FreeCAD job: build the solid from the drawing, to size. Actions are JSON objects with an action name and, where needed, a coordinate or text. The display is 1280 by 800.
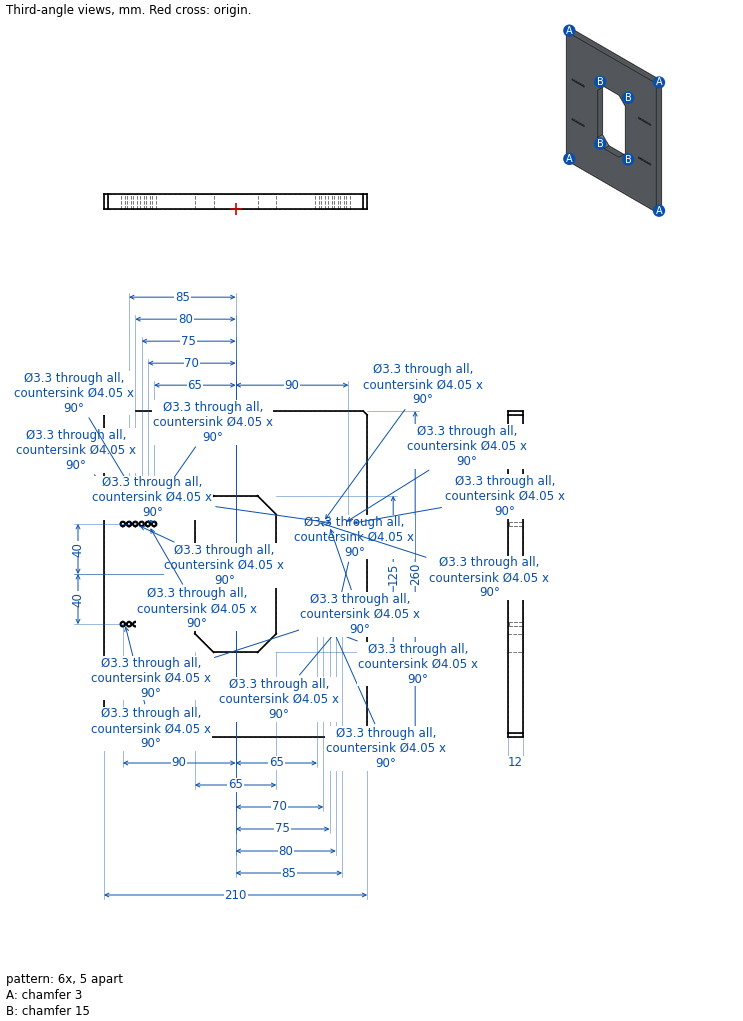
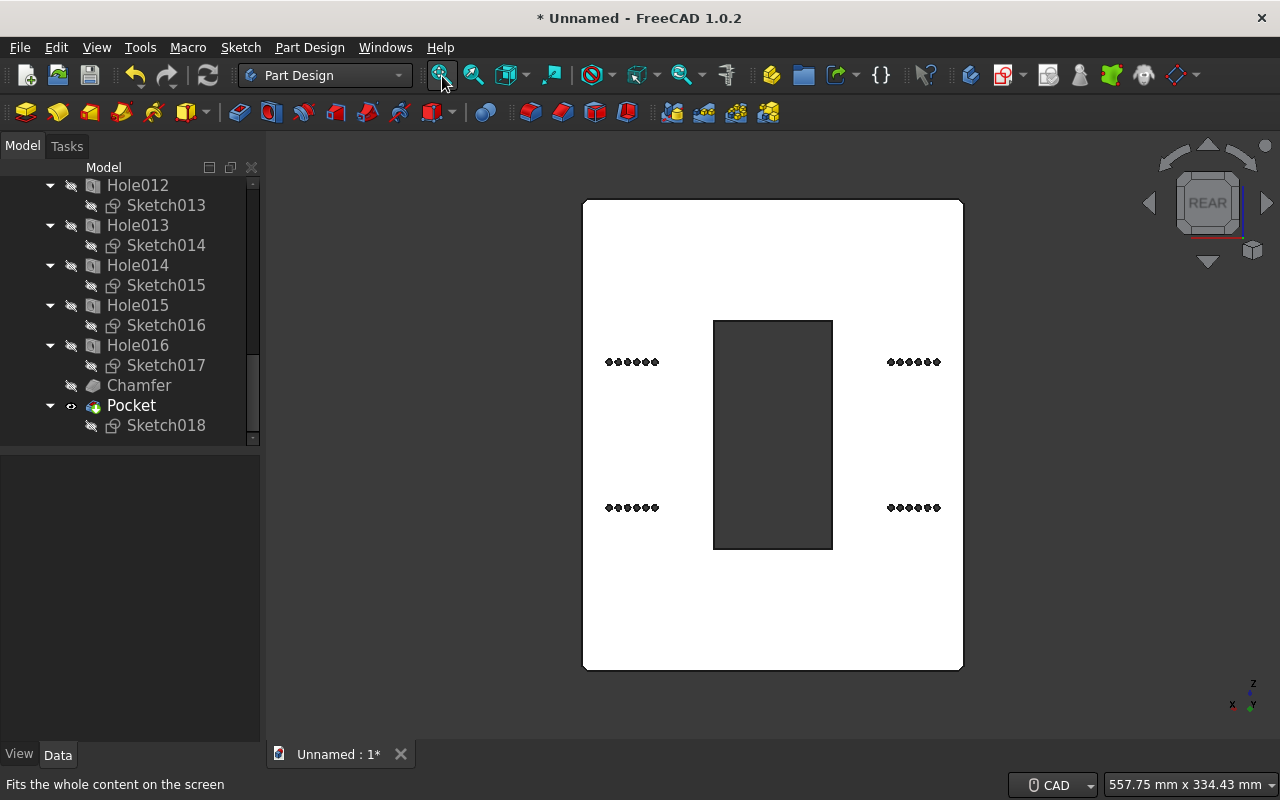
{"action": "scroll", "coordinate": [832, 548], "scroll_direction": "up", "scroll_amount": 4}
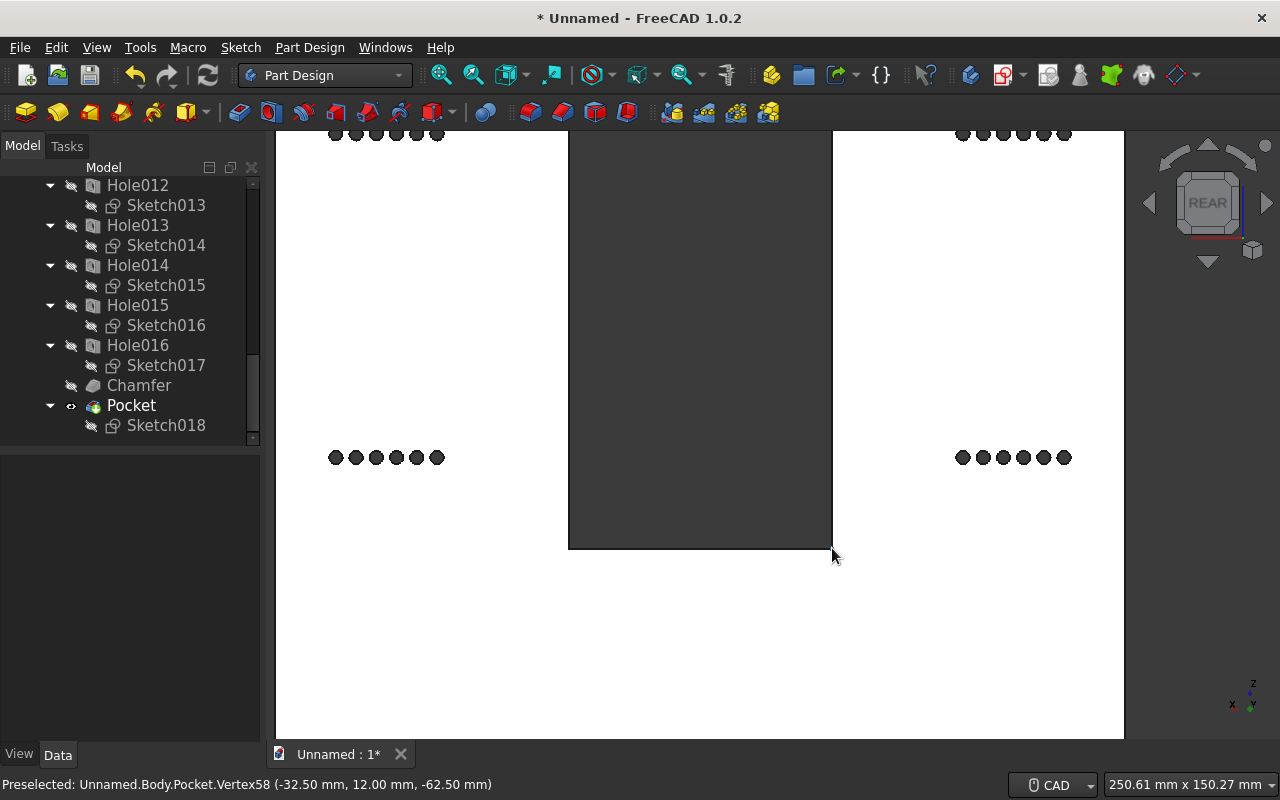
{"action": "left_click", "coordinate": [442, 76]}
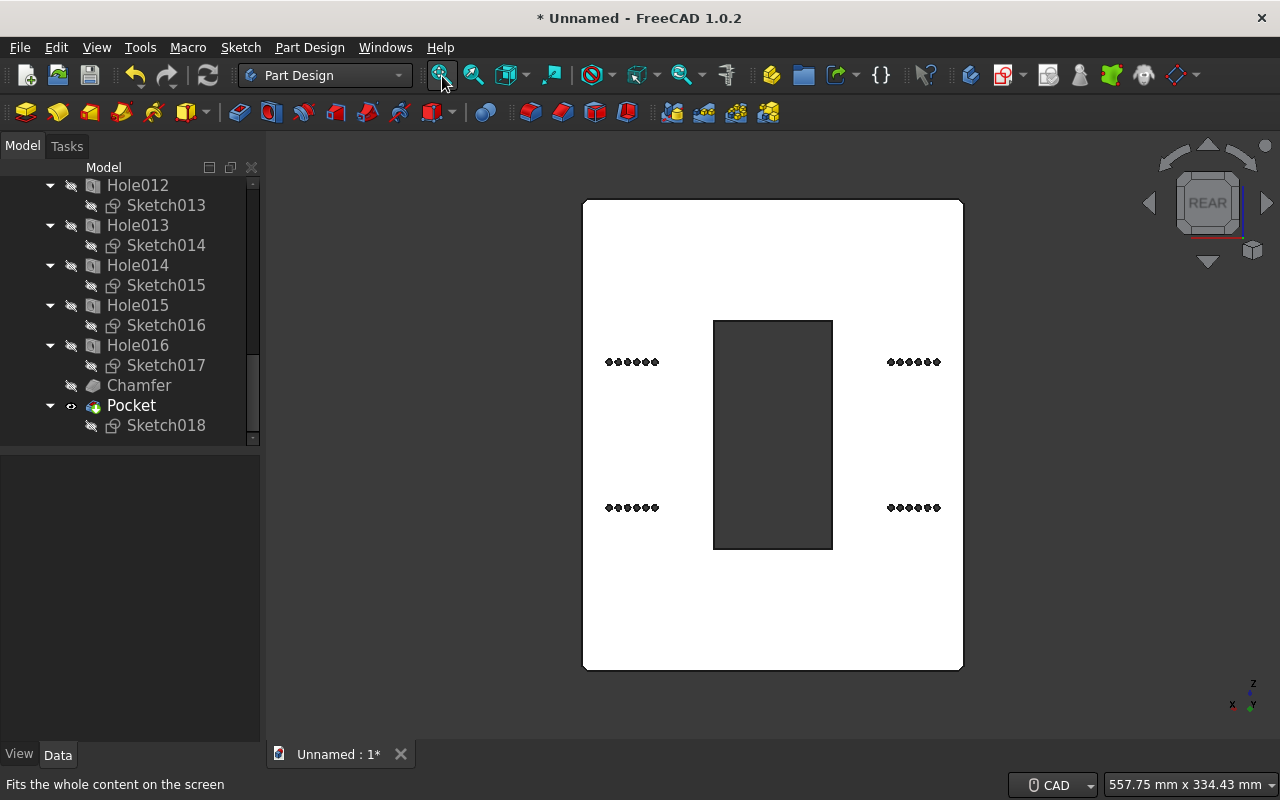
{"action": "key", "text": "6"}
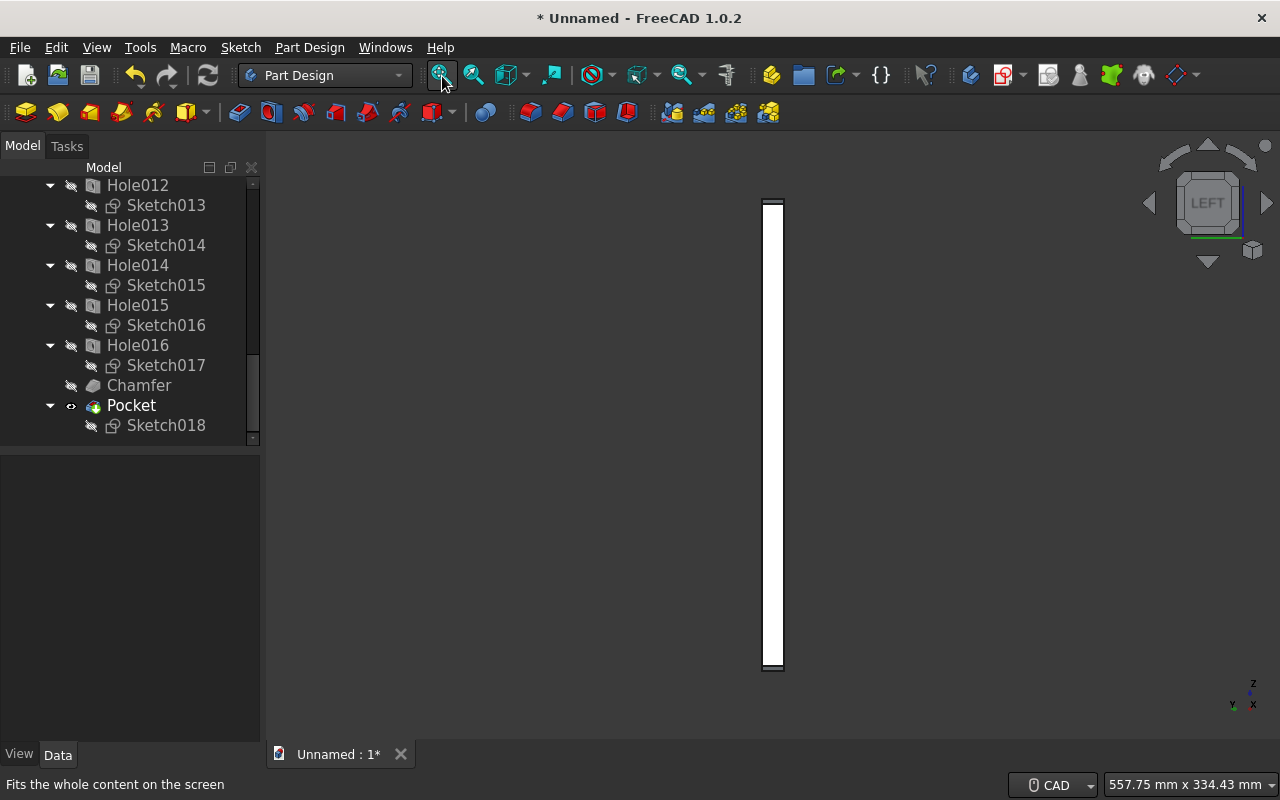
{"action": "scroll", "coordinate": [773, 548], "scroll_direction": "up", "scroll_amount": 4}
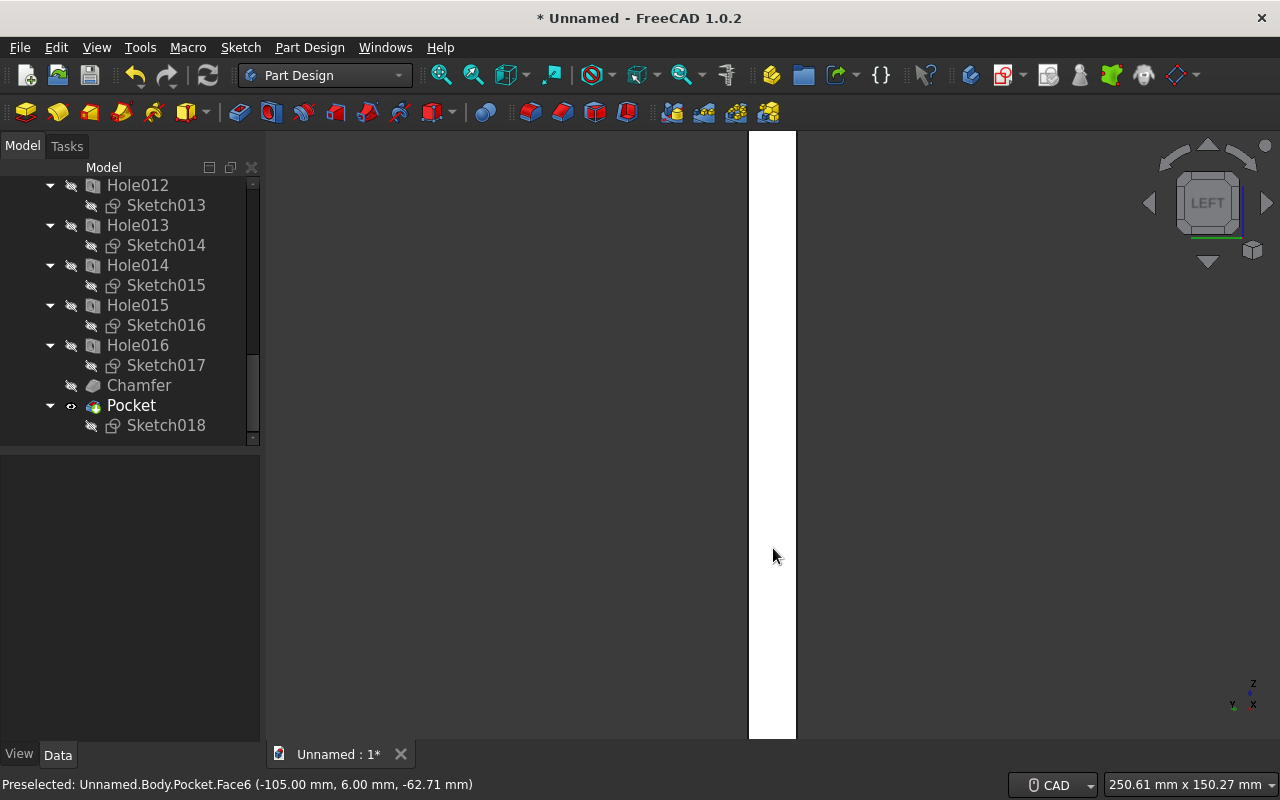
{"action": "left_click", "coordinate": [442, 76]}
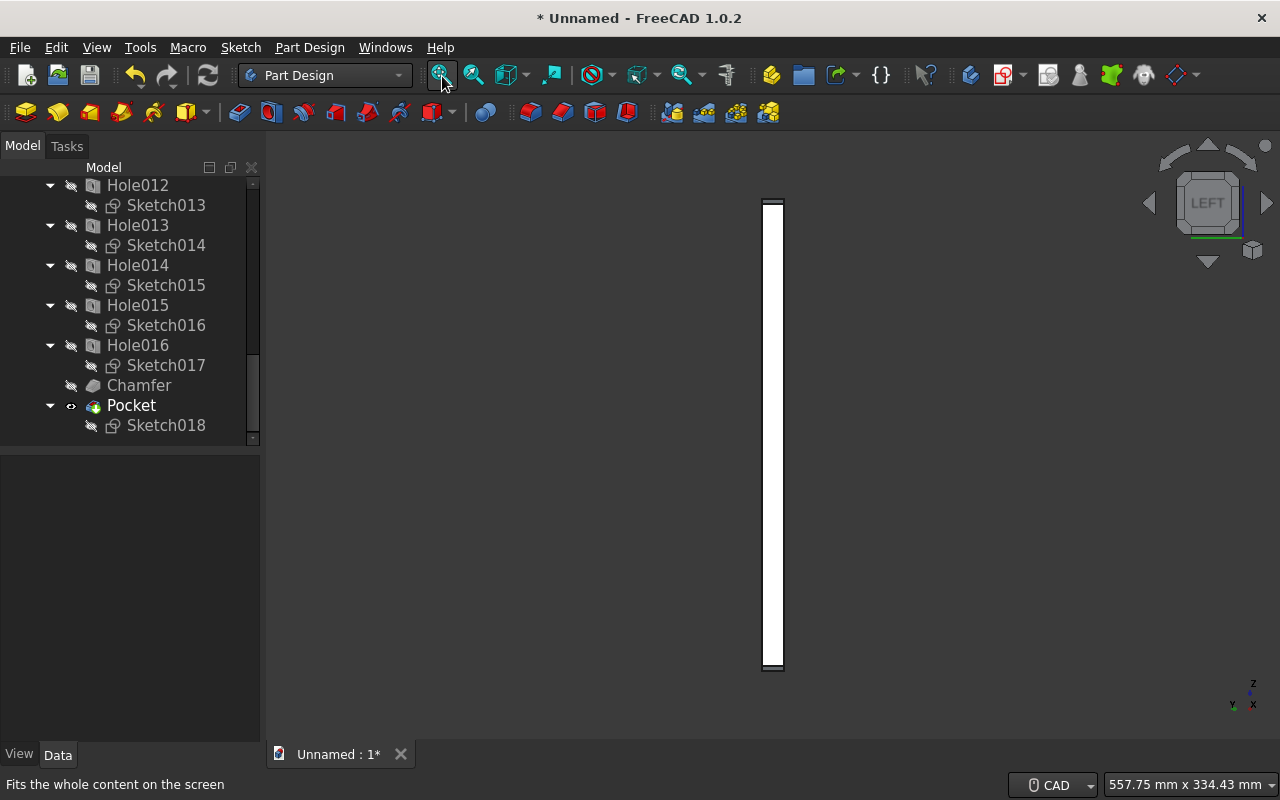
{"action": "key", "text": "v 3"}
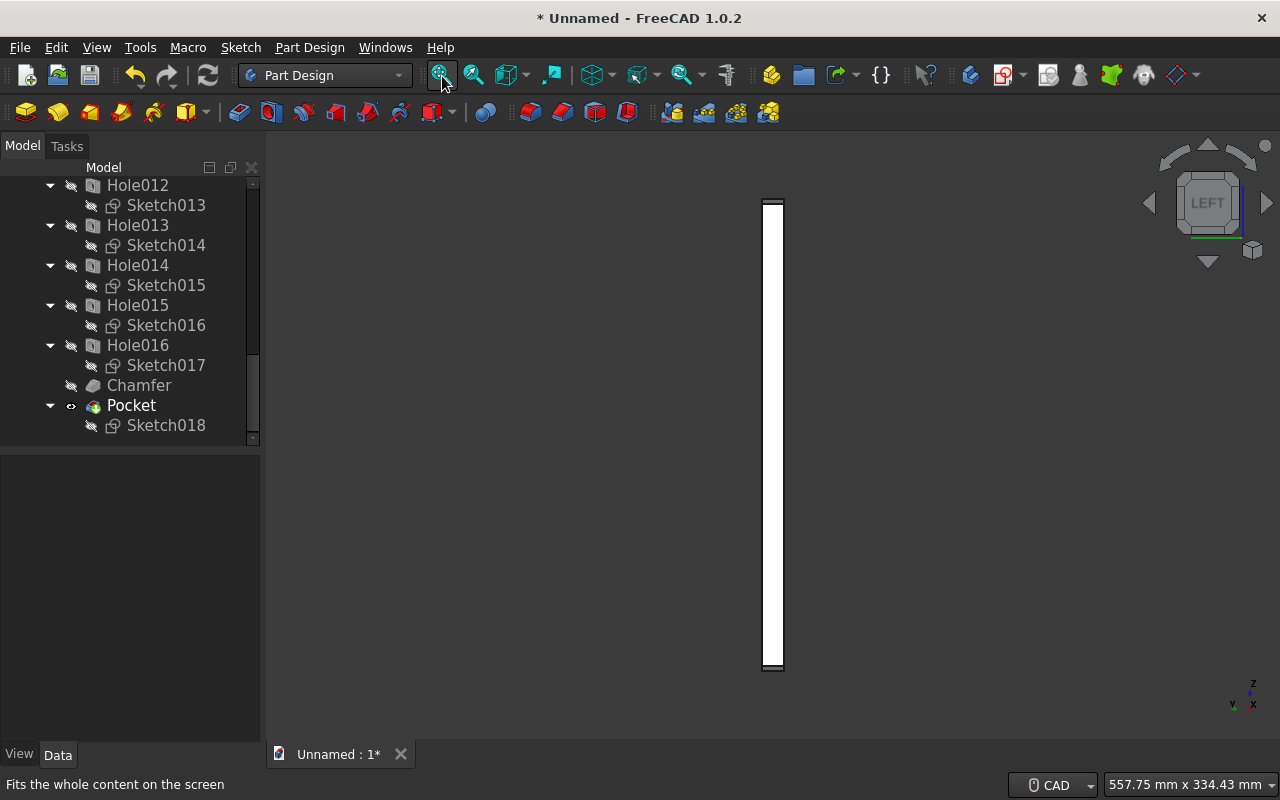
{"action": "key", "text": "0"}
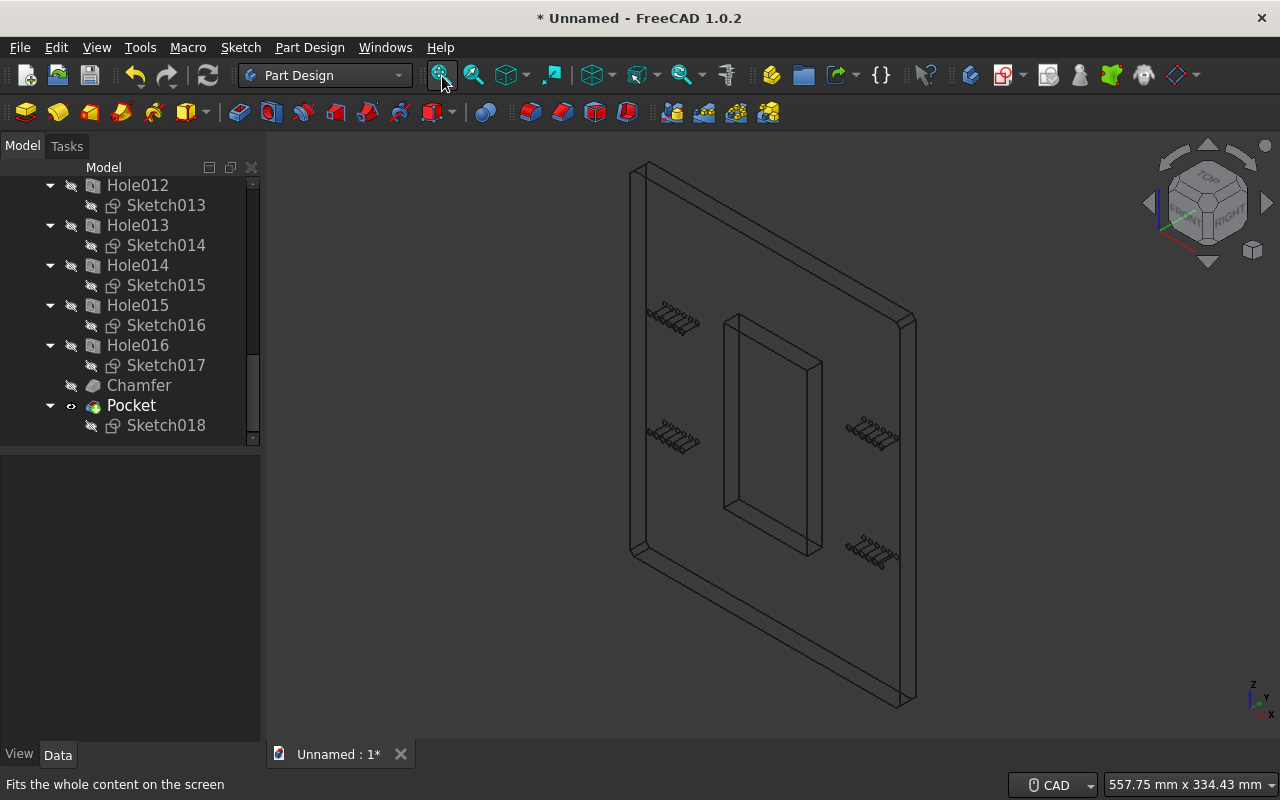
{"action": "left_click", "coordinate": [731, 503]}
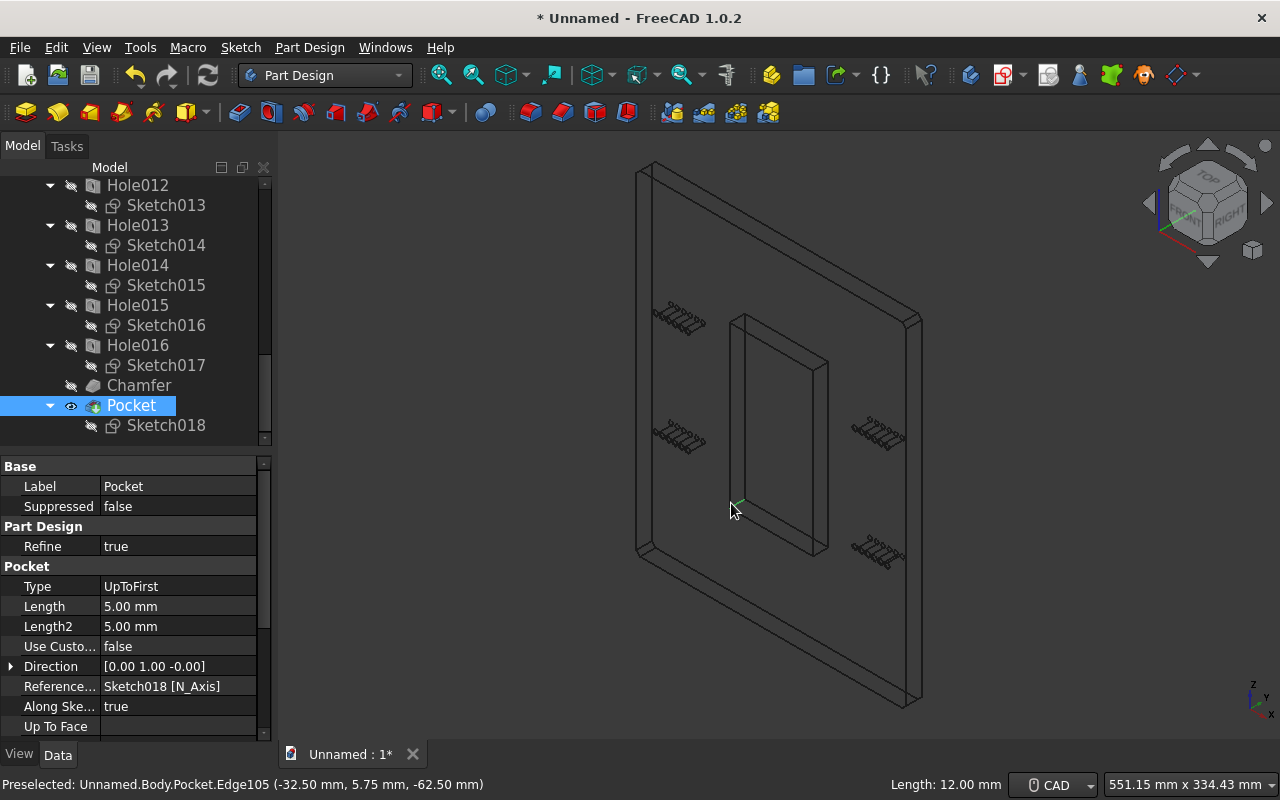
{"action": "left_click", "coordinate": [737, 317], "text": "ctrl"}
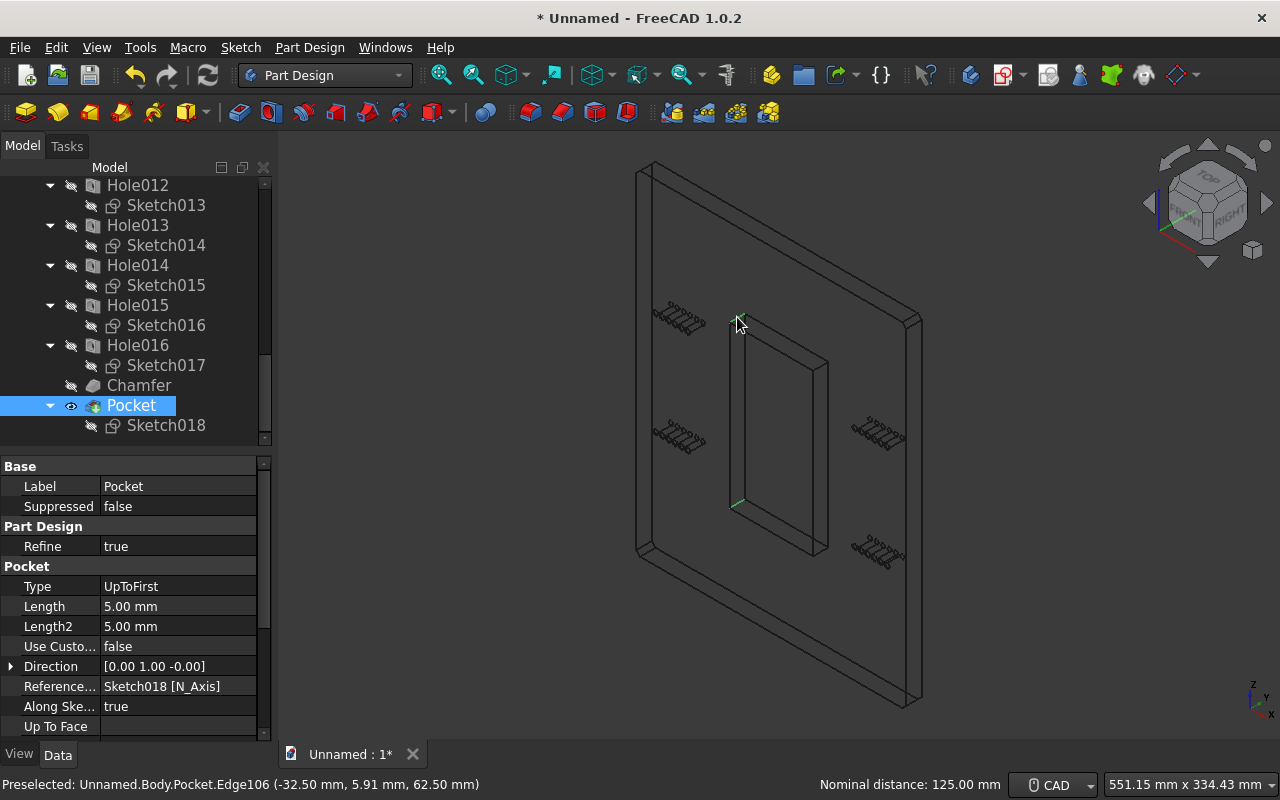
{"action": "left_click", "coordinate": [821, 365], "text": "ctrl"}